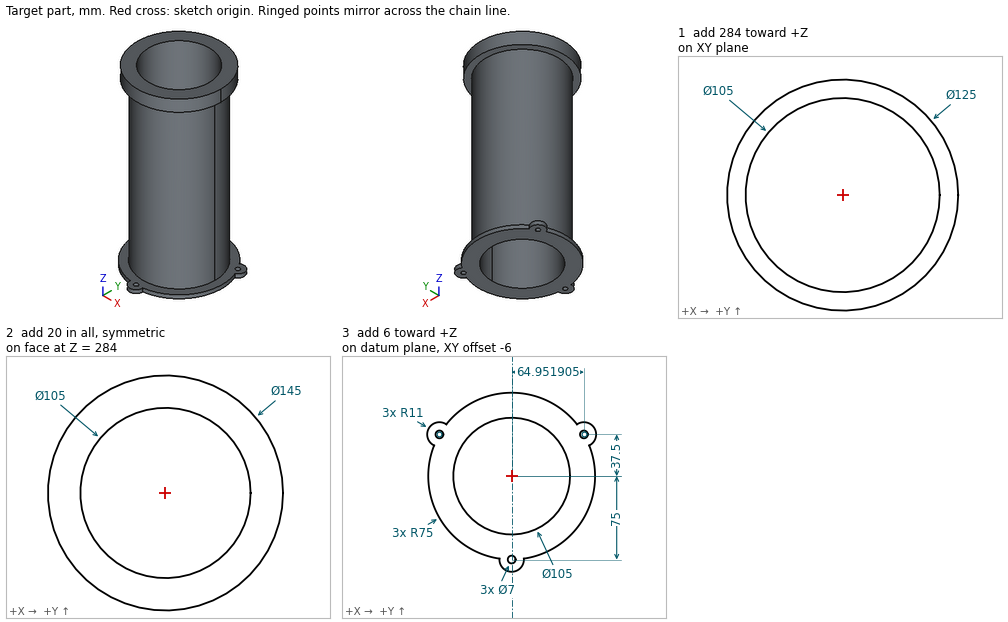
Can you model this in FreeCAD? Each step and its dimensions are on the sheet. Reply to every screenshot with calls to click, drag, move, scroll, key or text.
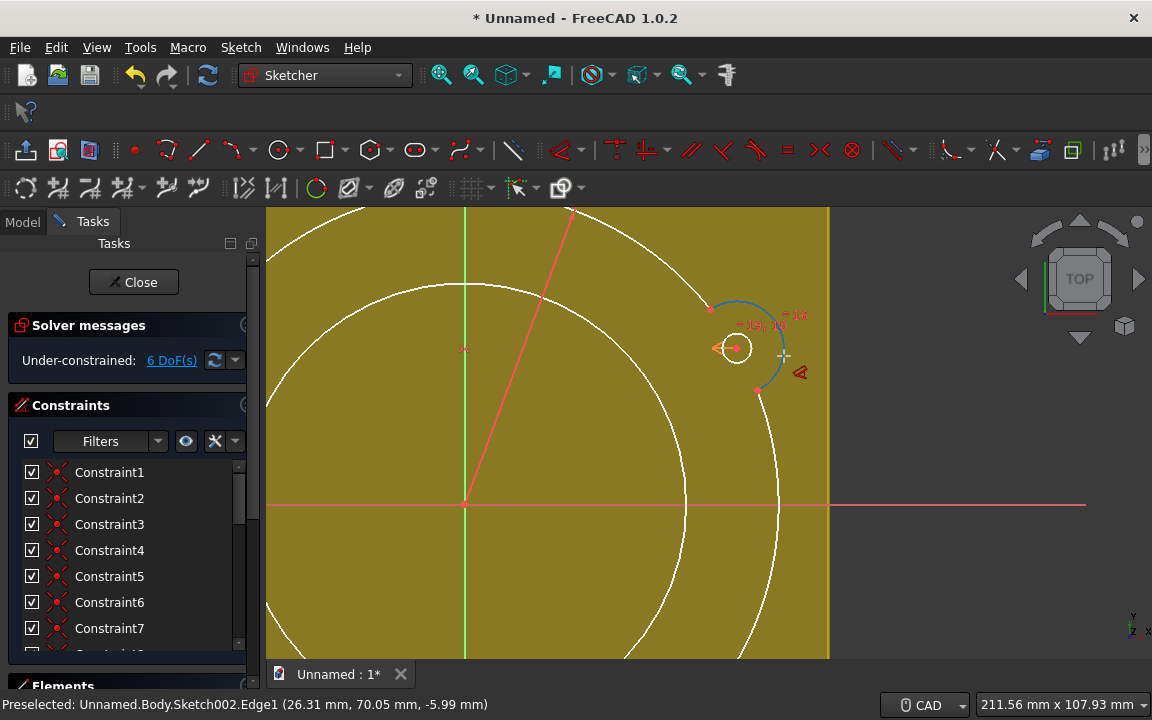
click(783, 355)
click(815, 360)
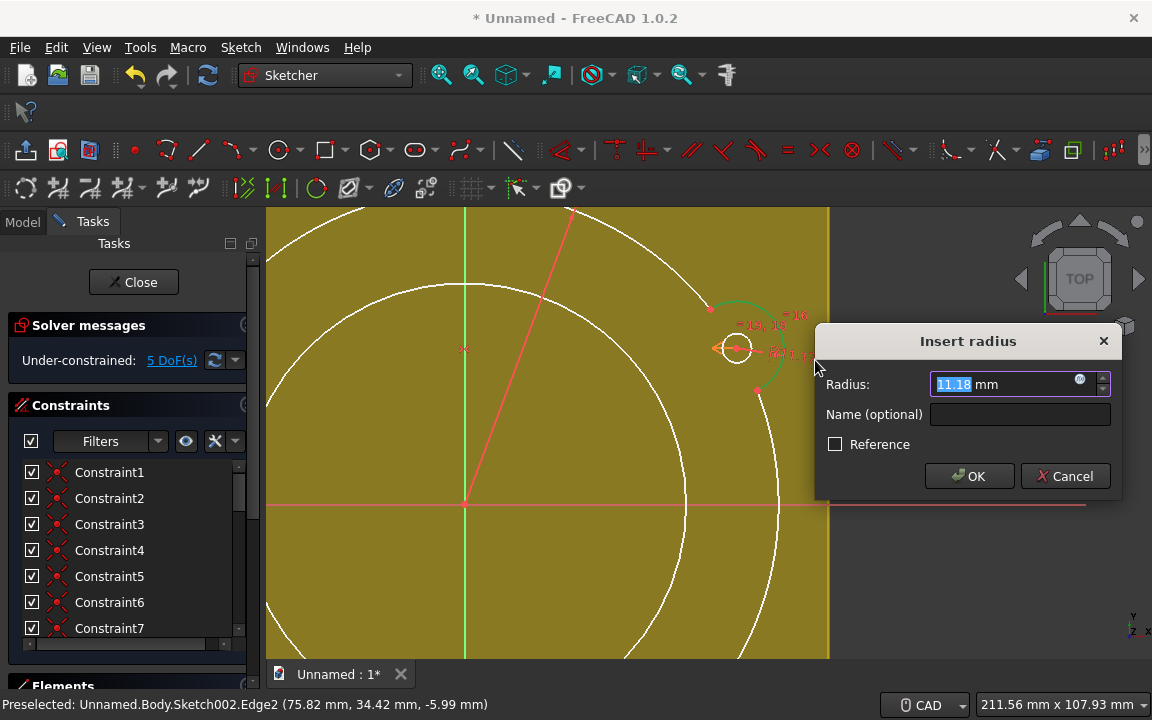
text(11)
key(Return)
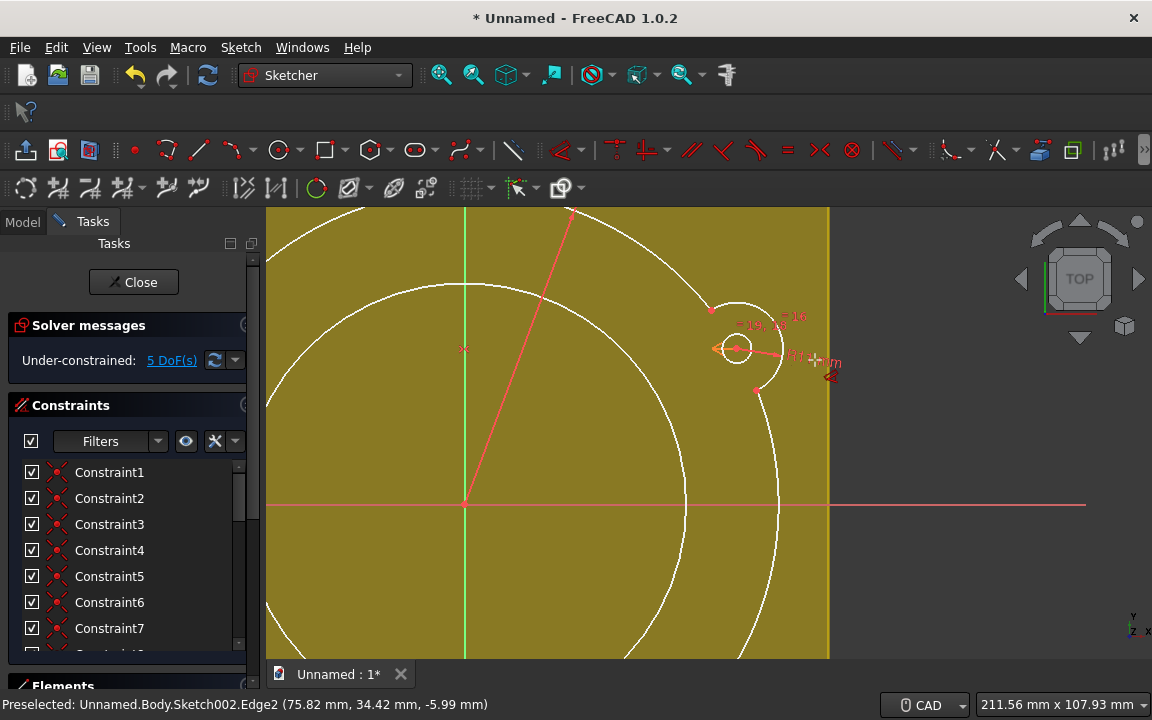
scroll(784, 356, down, 4)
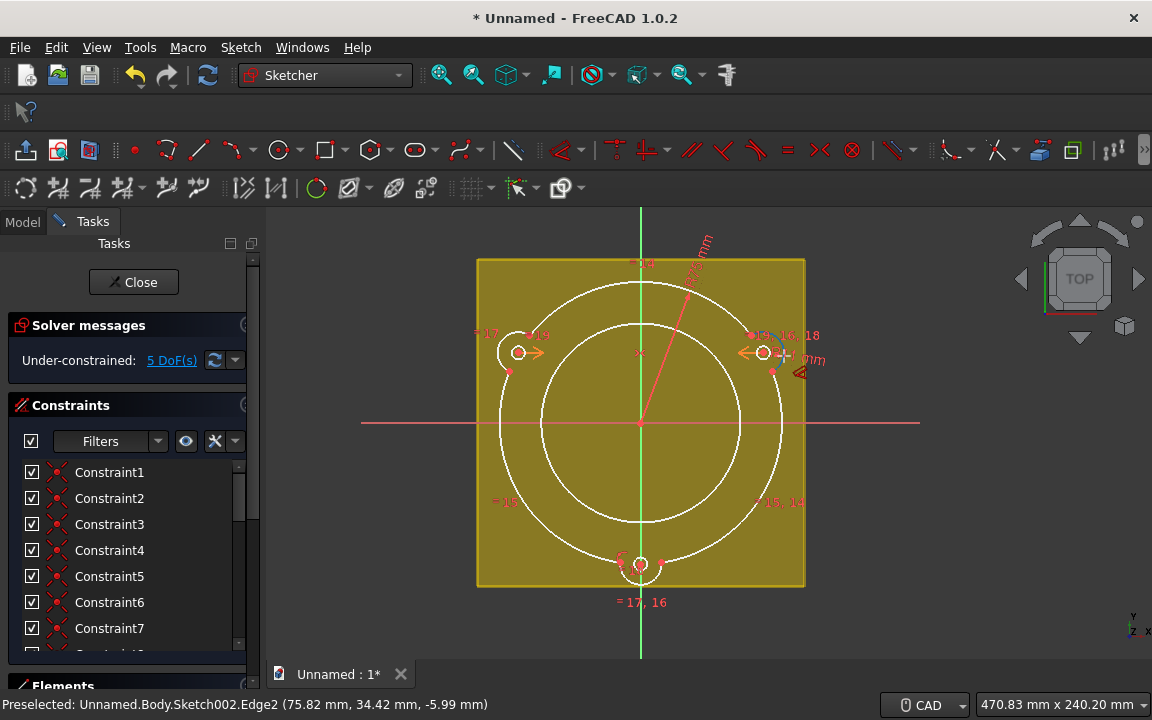
scroll(645, 559, up, 6)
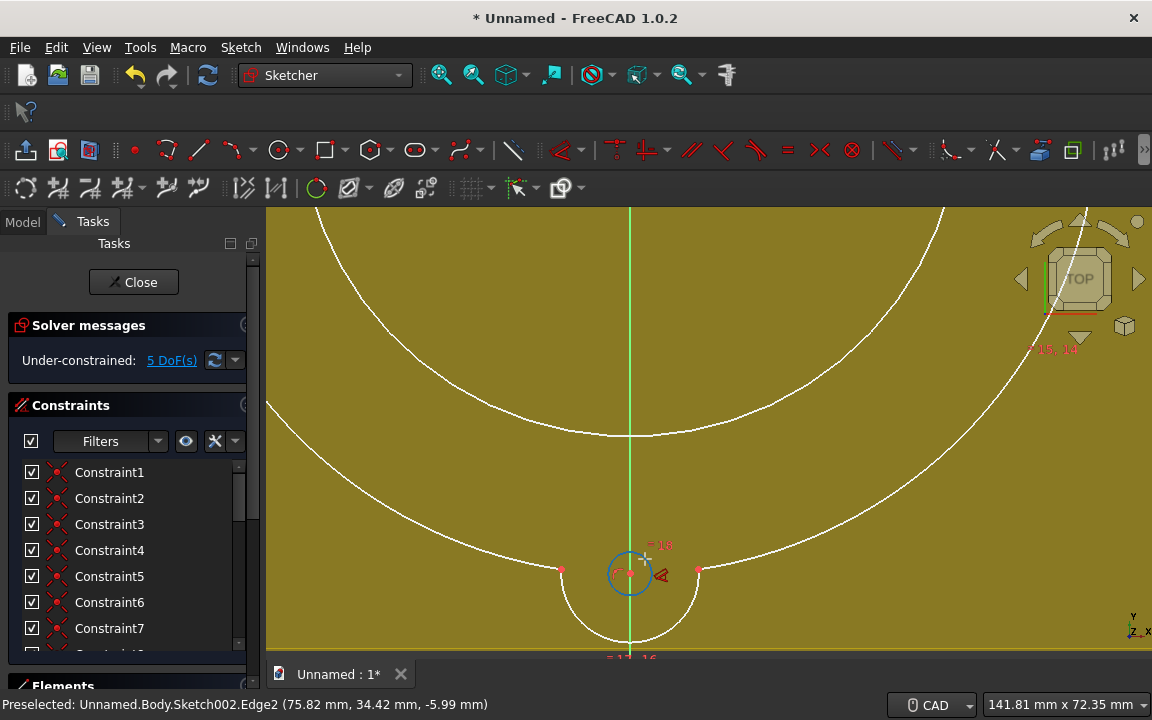
click(645, 558)
click(667, 535)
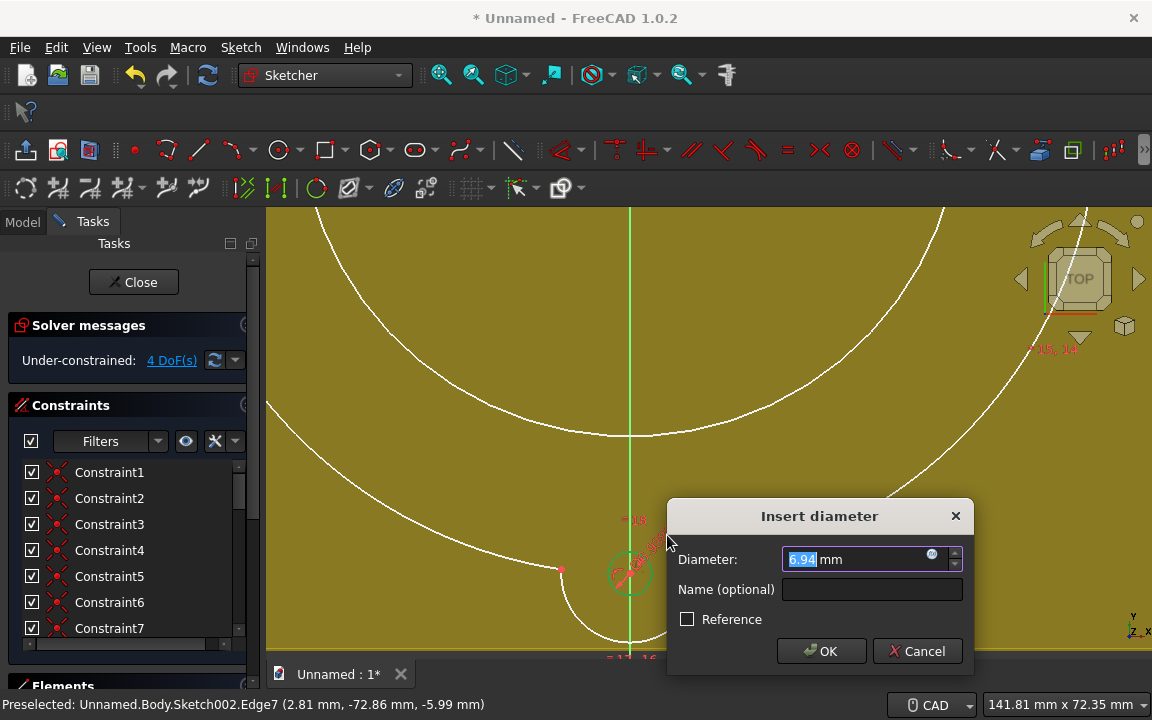
text(7)
key(Return)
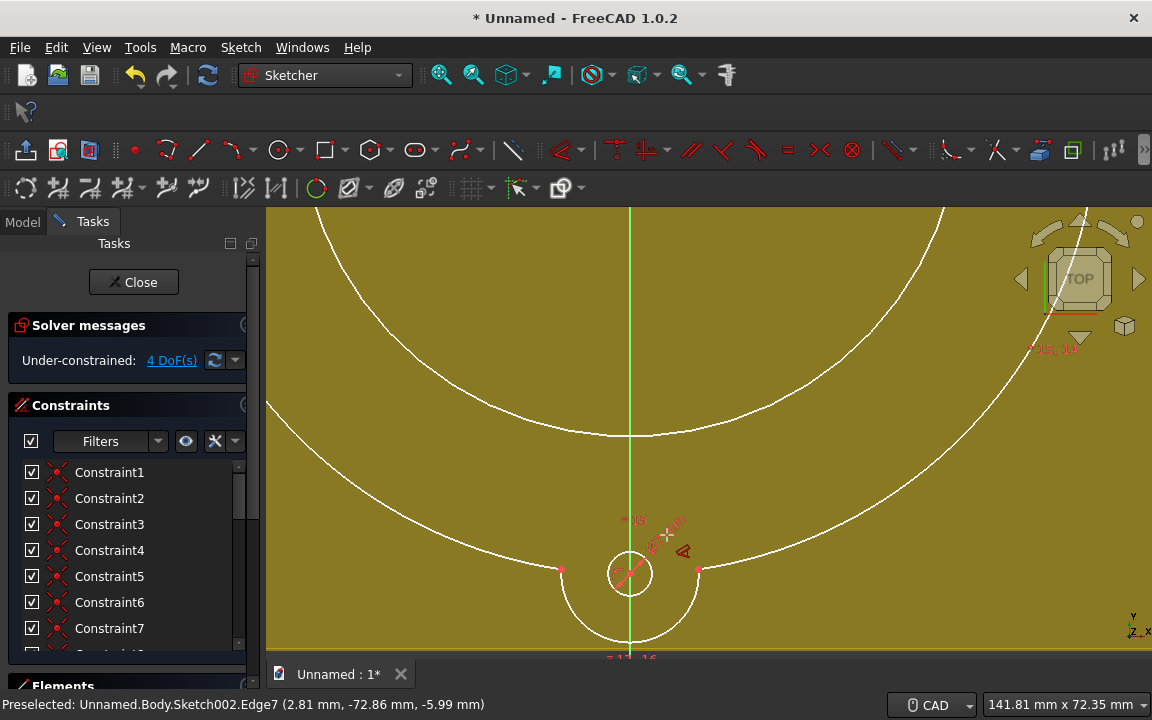
click(397, 340)
click(374, 363)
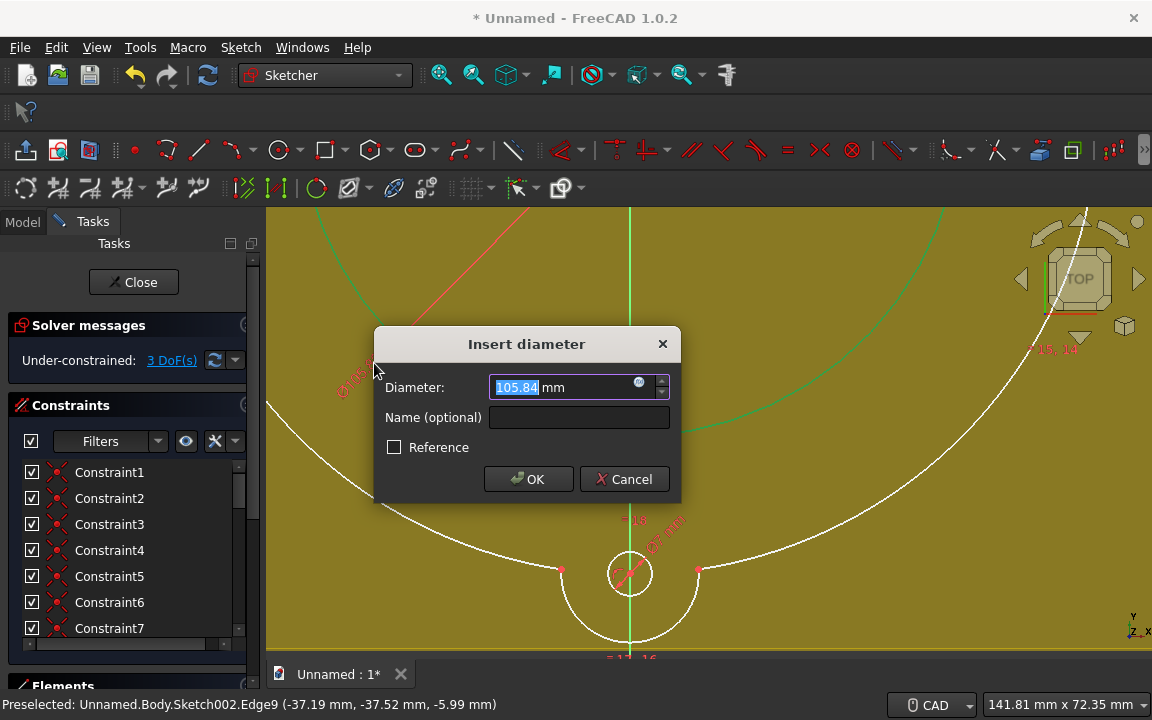
text(105)
key(Return)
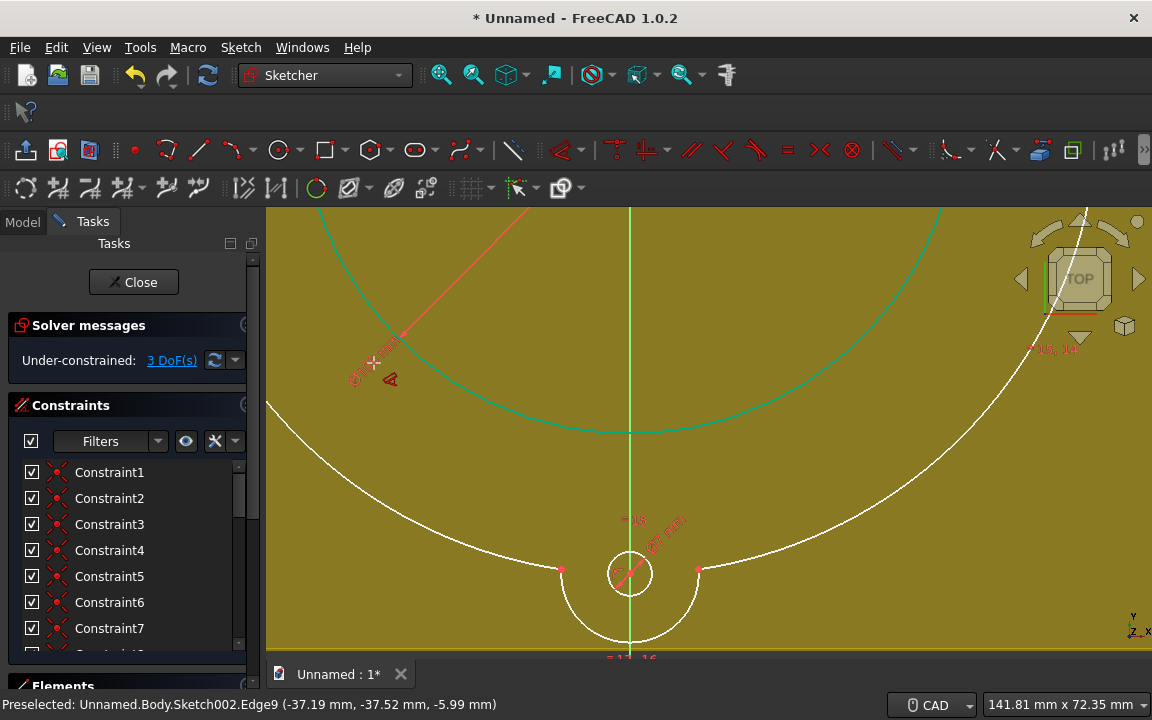
click(630, 574)
click(664, 404)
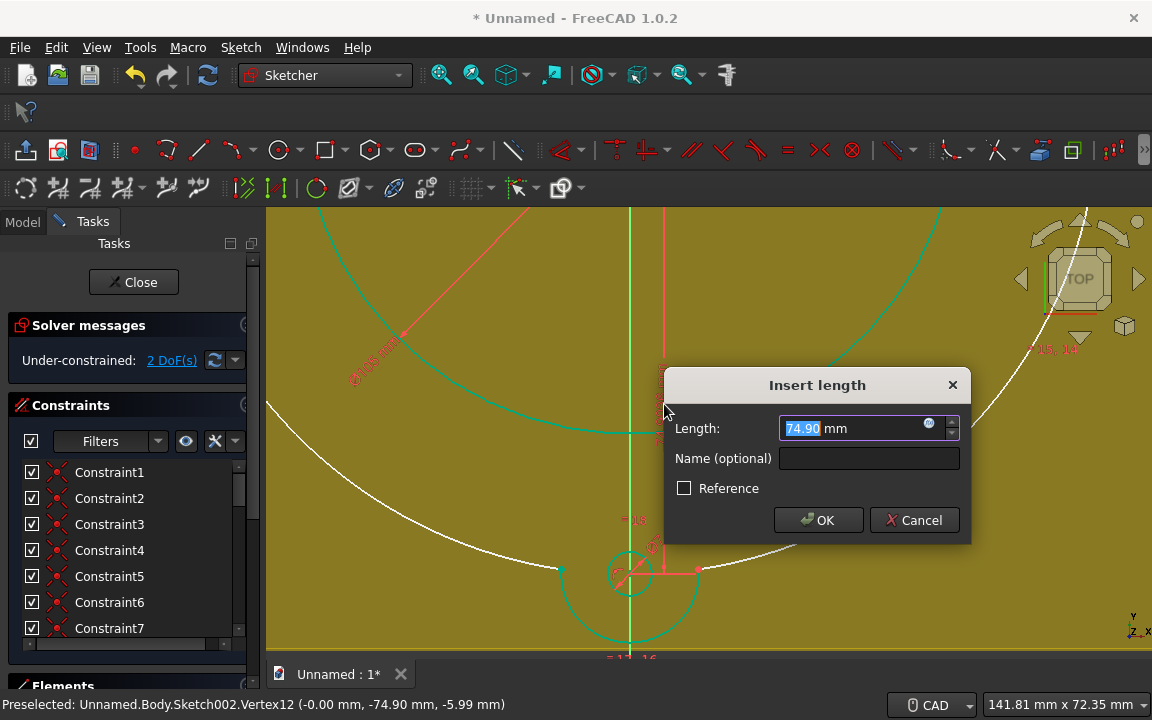
text(75)
key(Return)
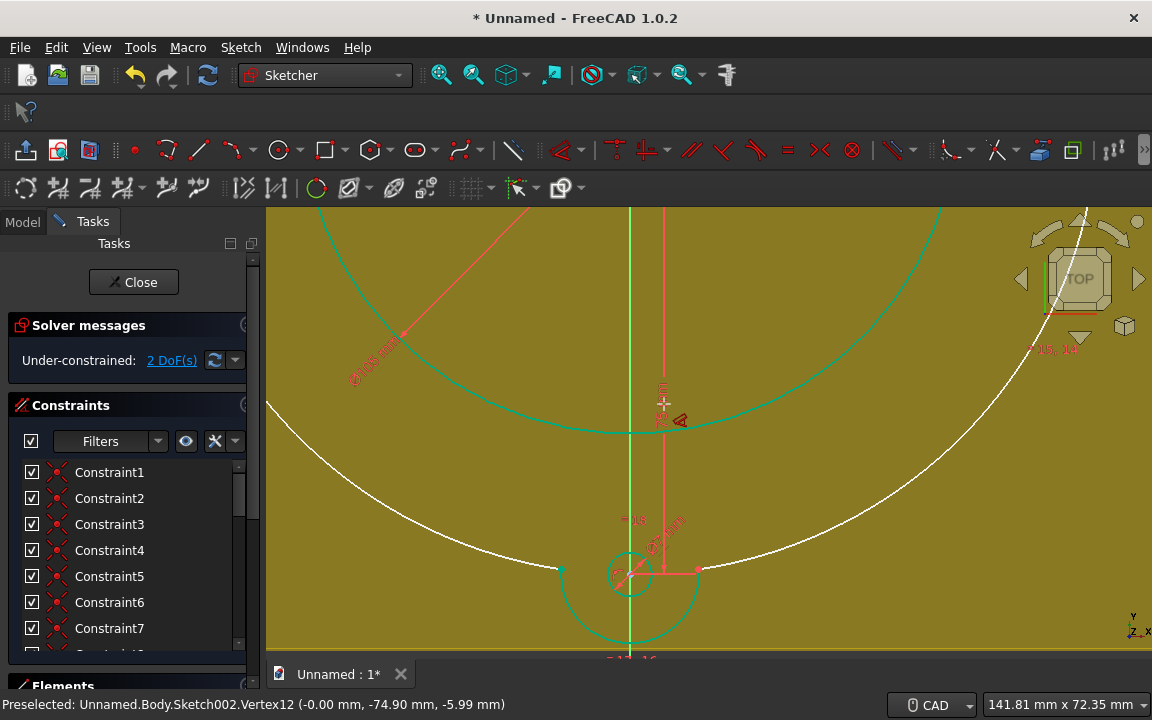
scroll(645, 559, down, 6)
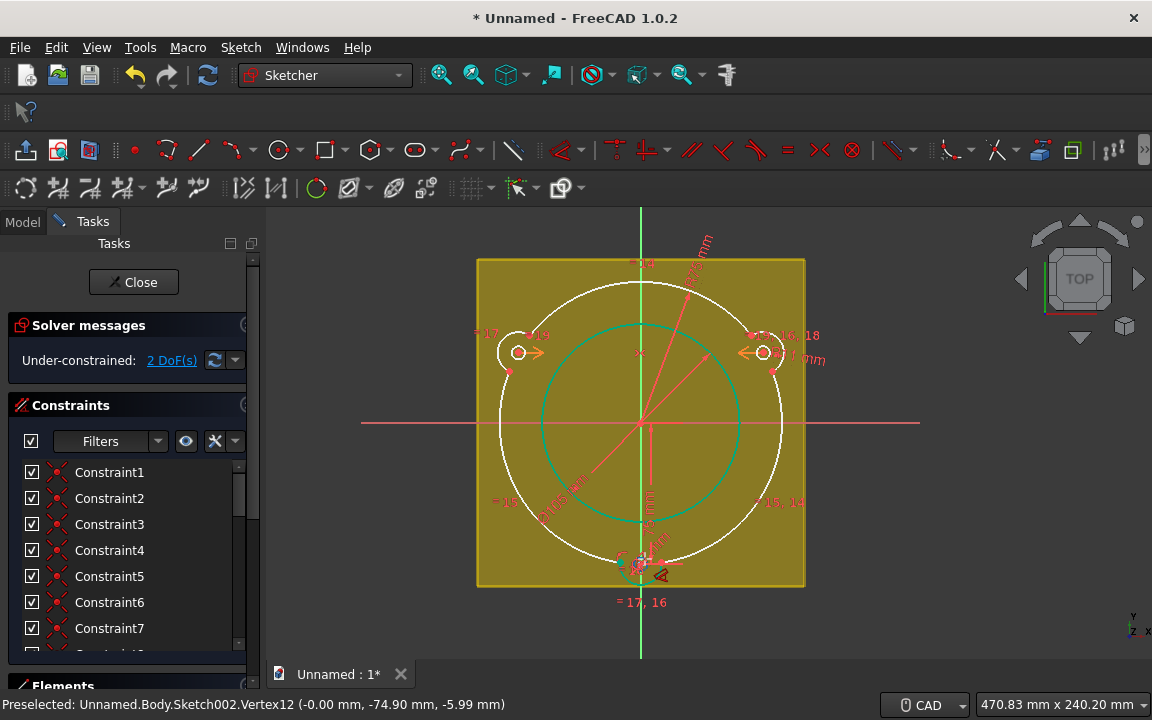
click(763, 353)
click(797, 388)